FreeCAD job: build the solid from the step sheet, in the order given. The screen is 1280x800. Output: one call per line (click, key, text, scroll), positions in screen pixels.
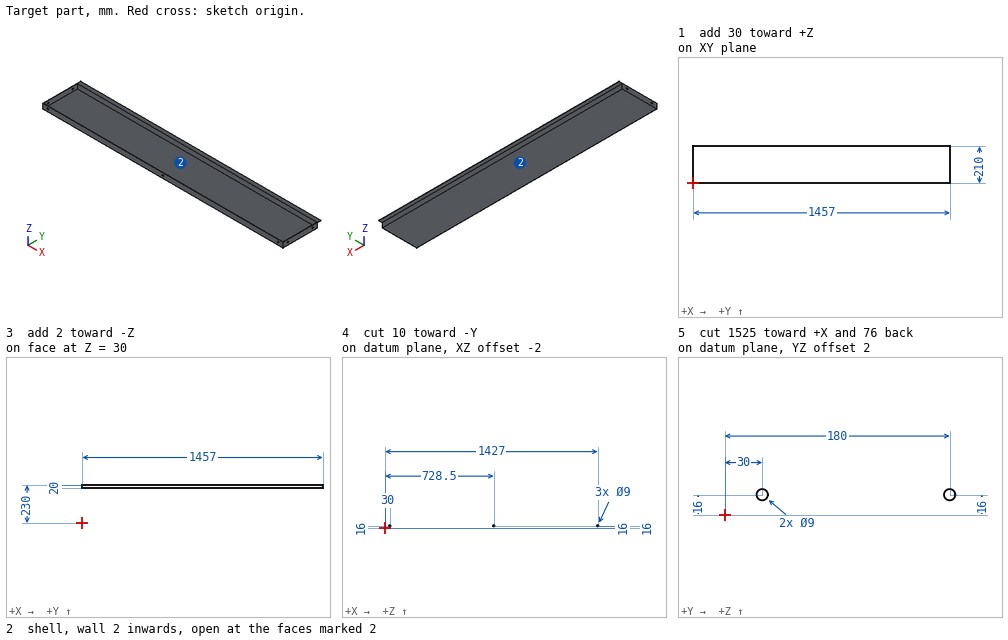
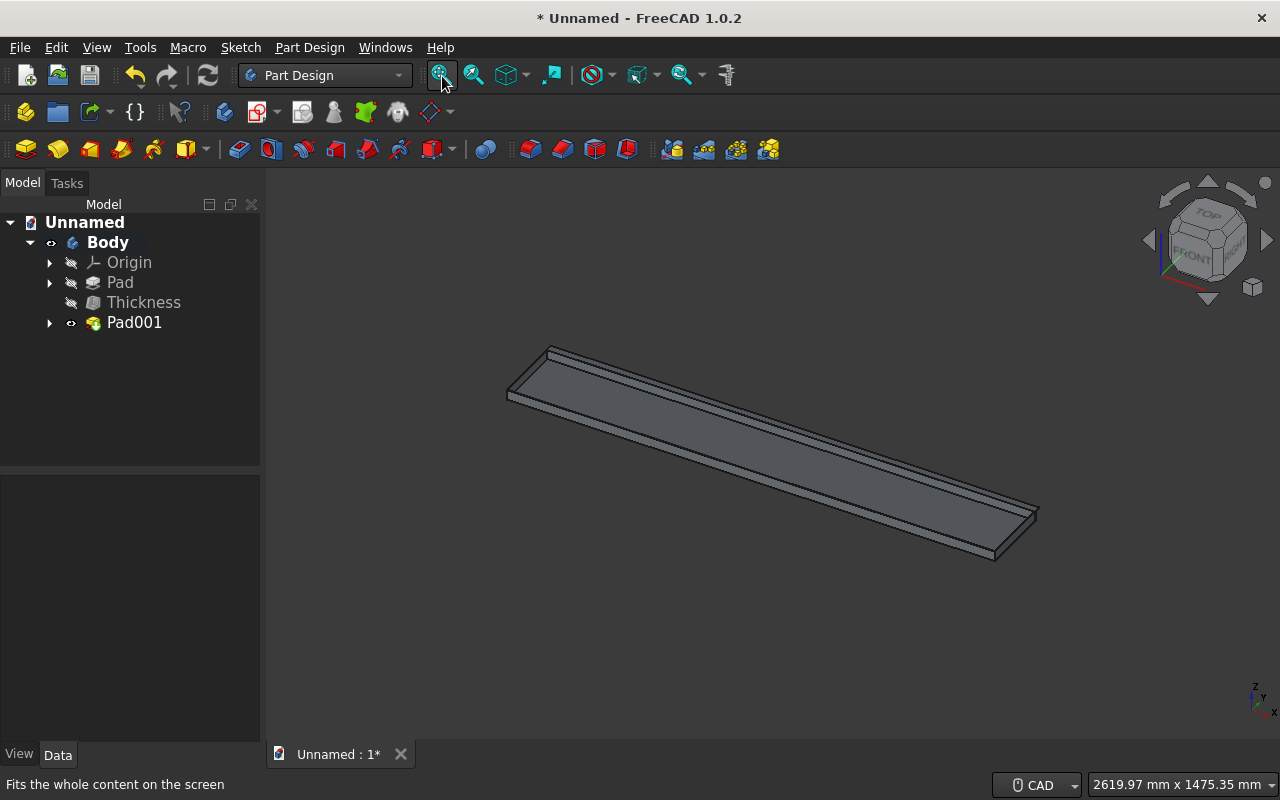
click(50, 263)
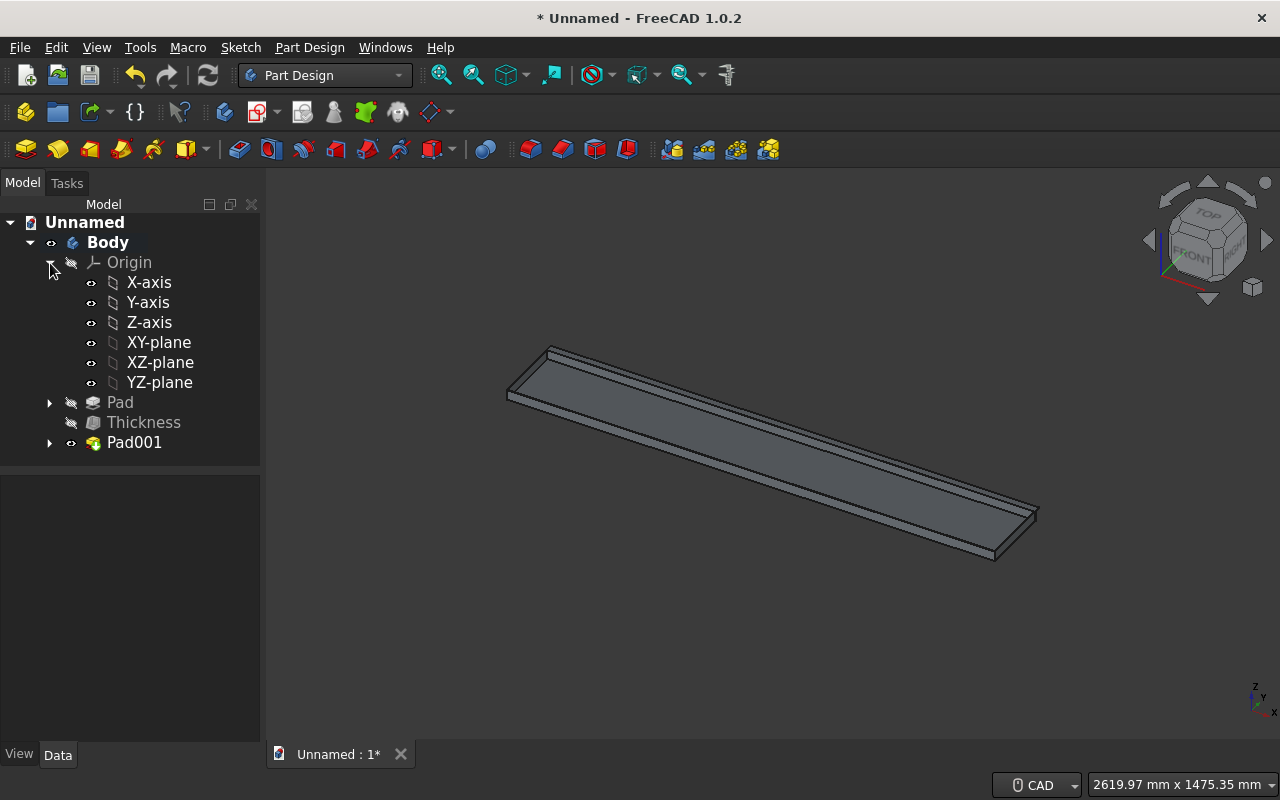
click(136, 363)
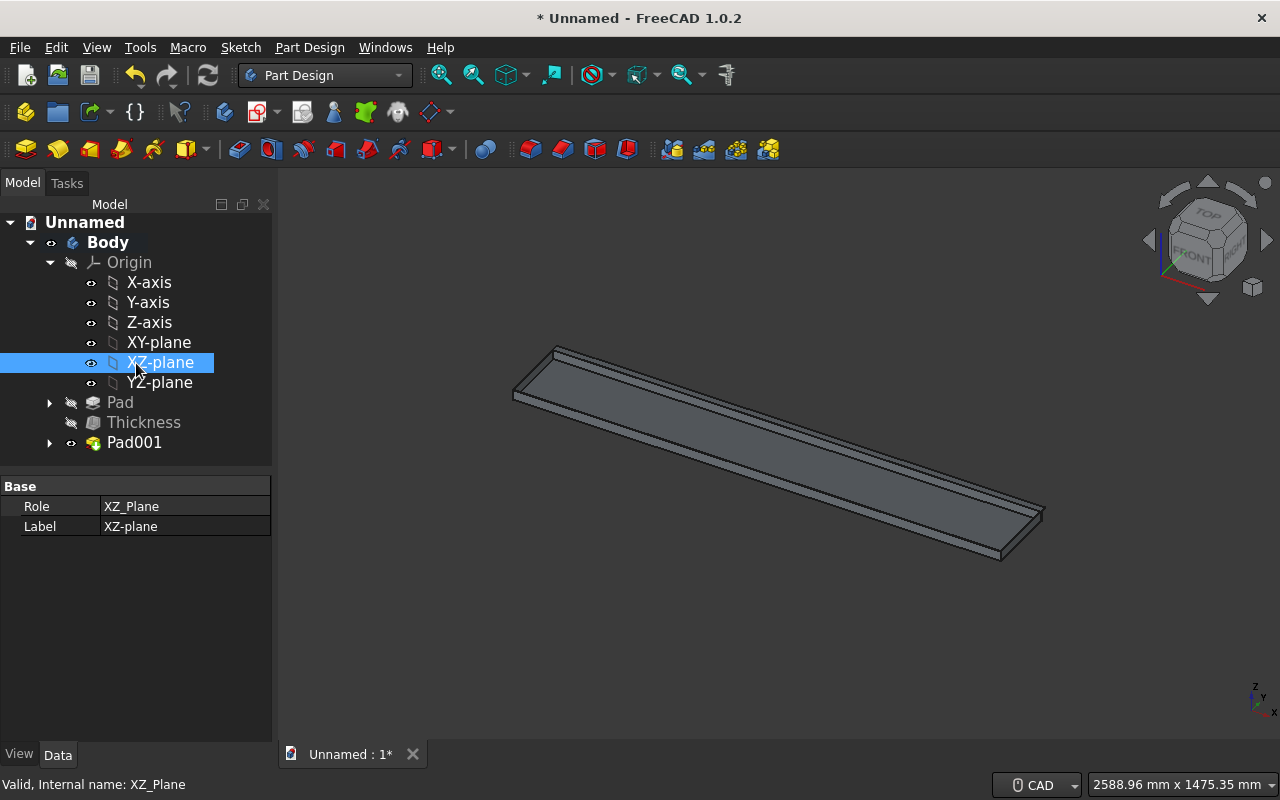
click(430, 112)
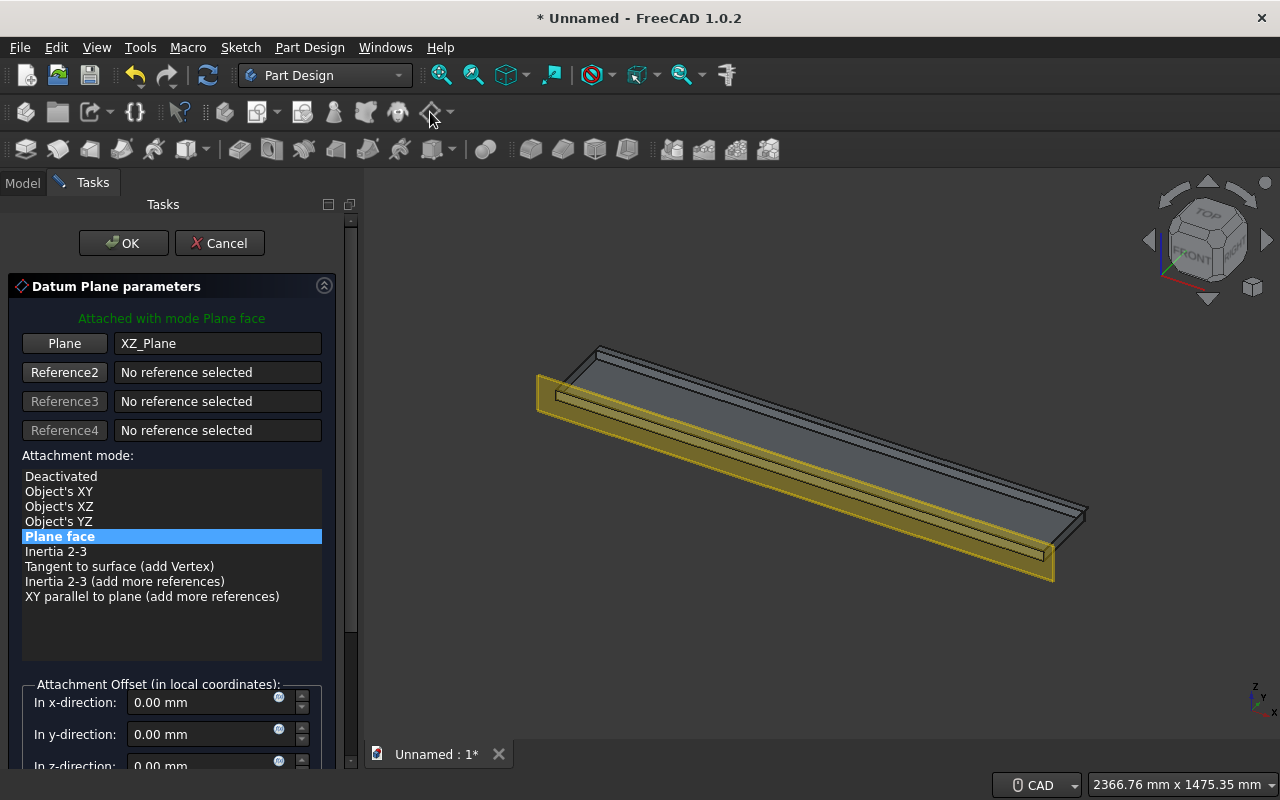
scroll(351, 491, down, 2)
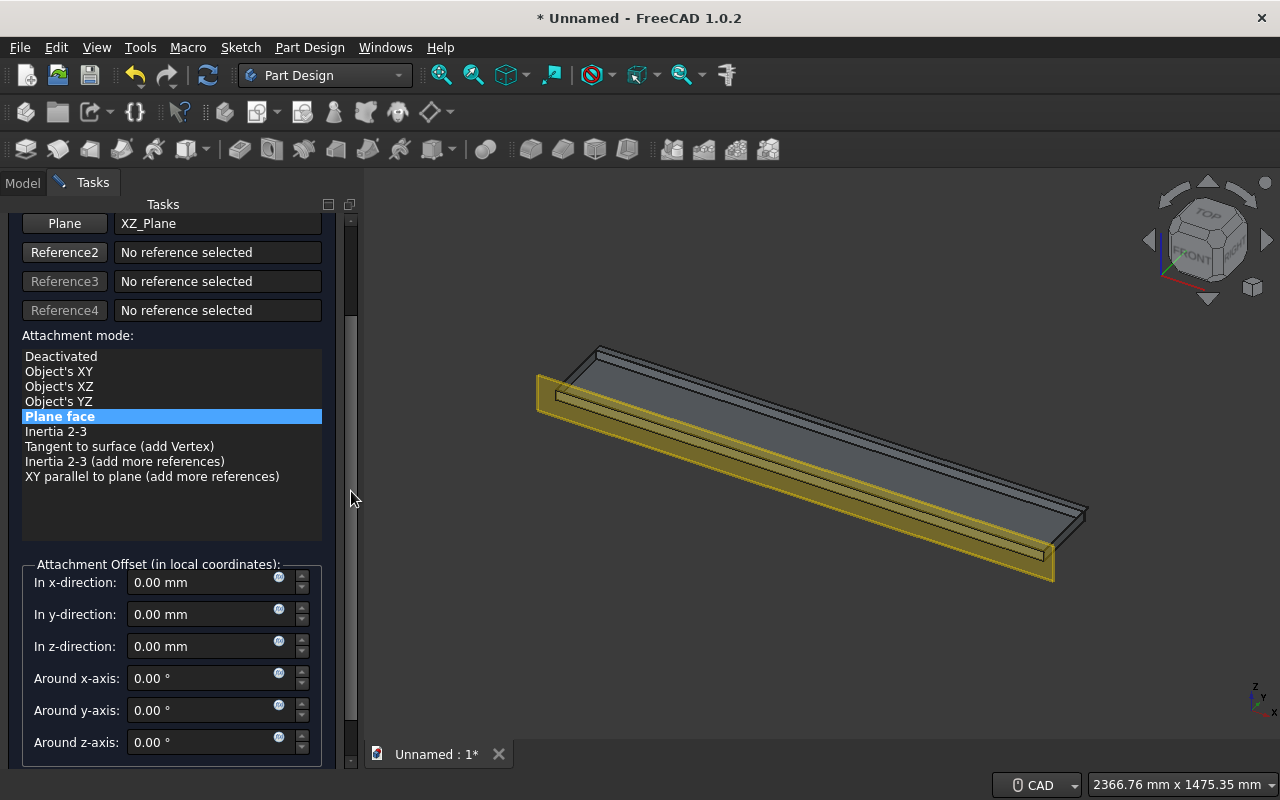
triple_click(210, 646)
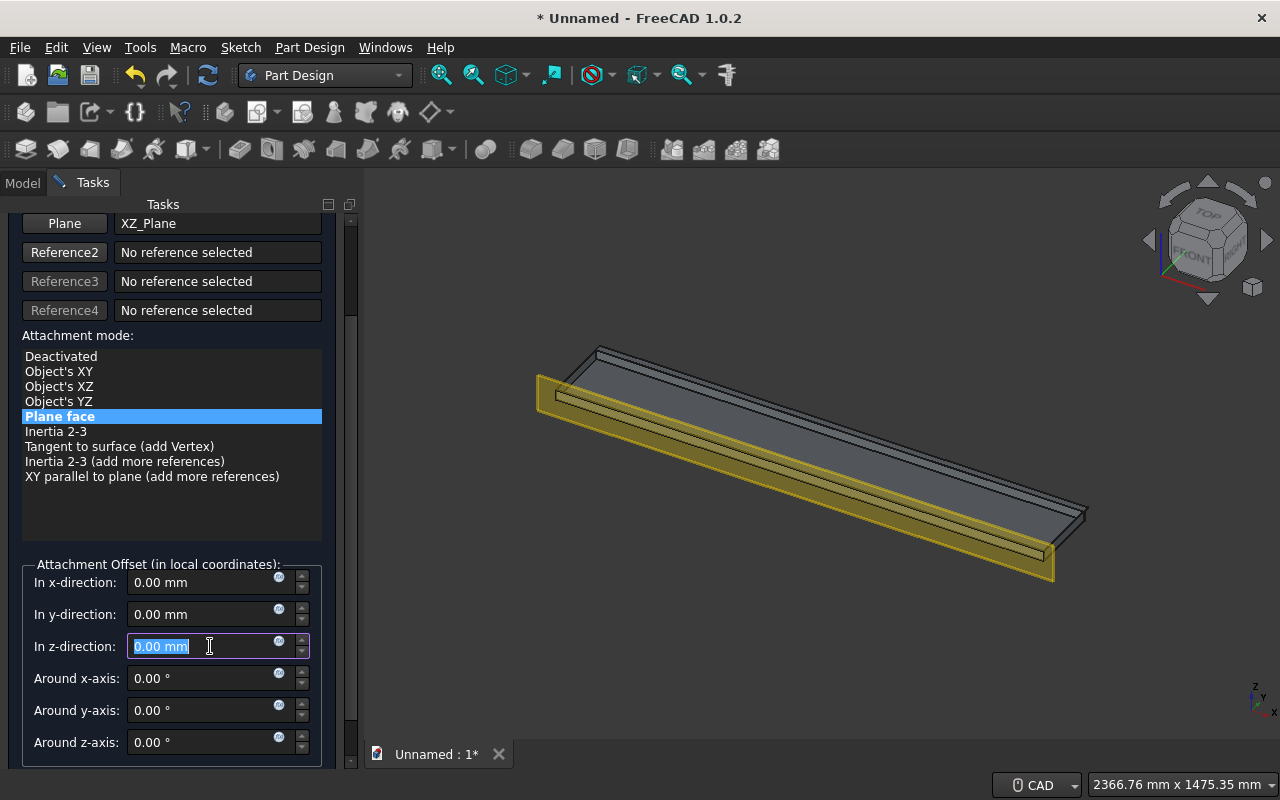
text(-2)
key(Tab)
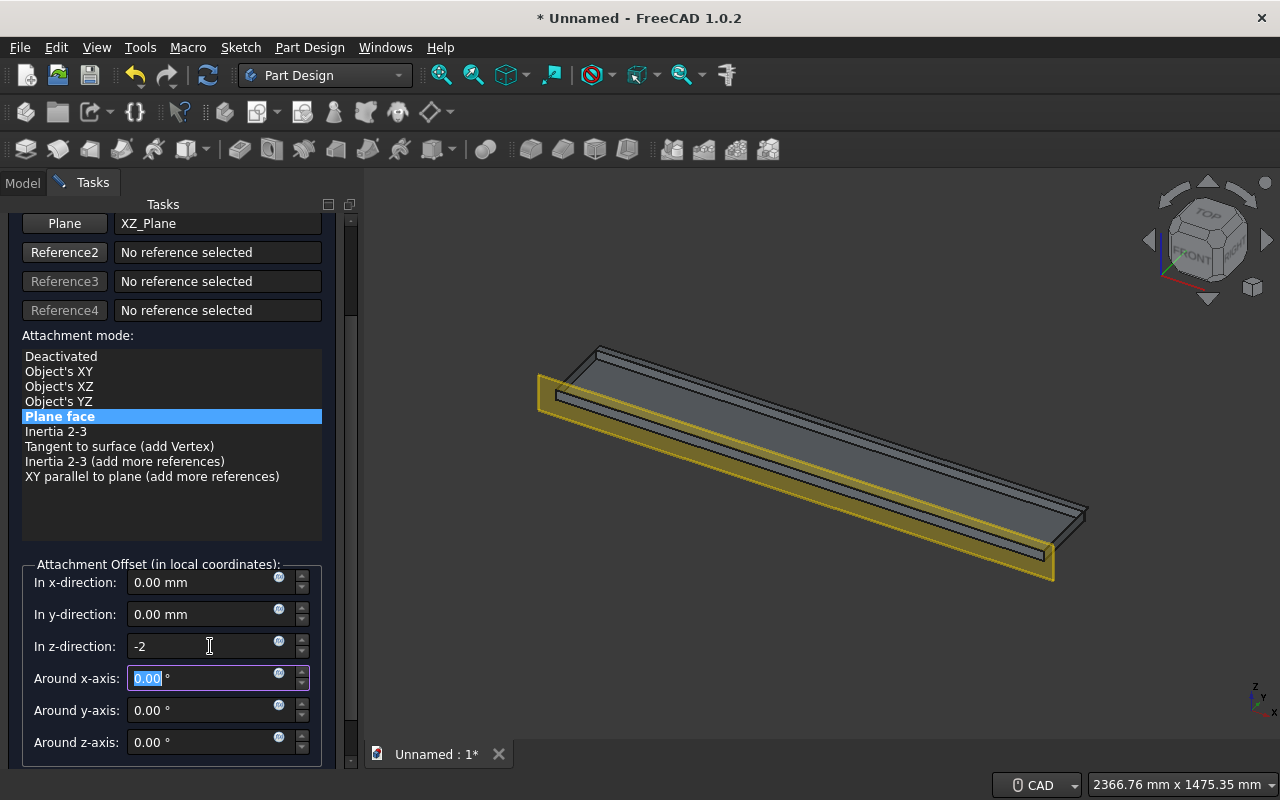
scroll(351, 491, up, 3)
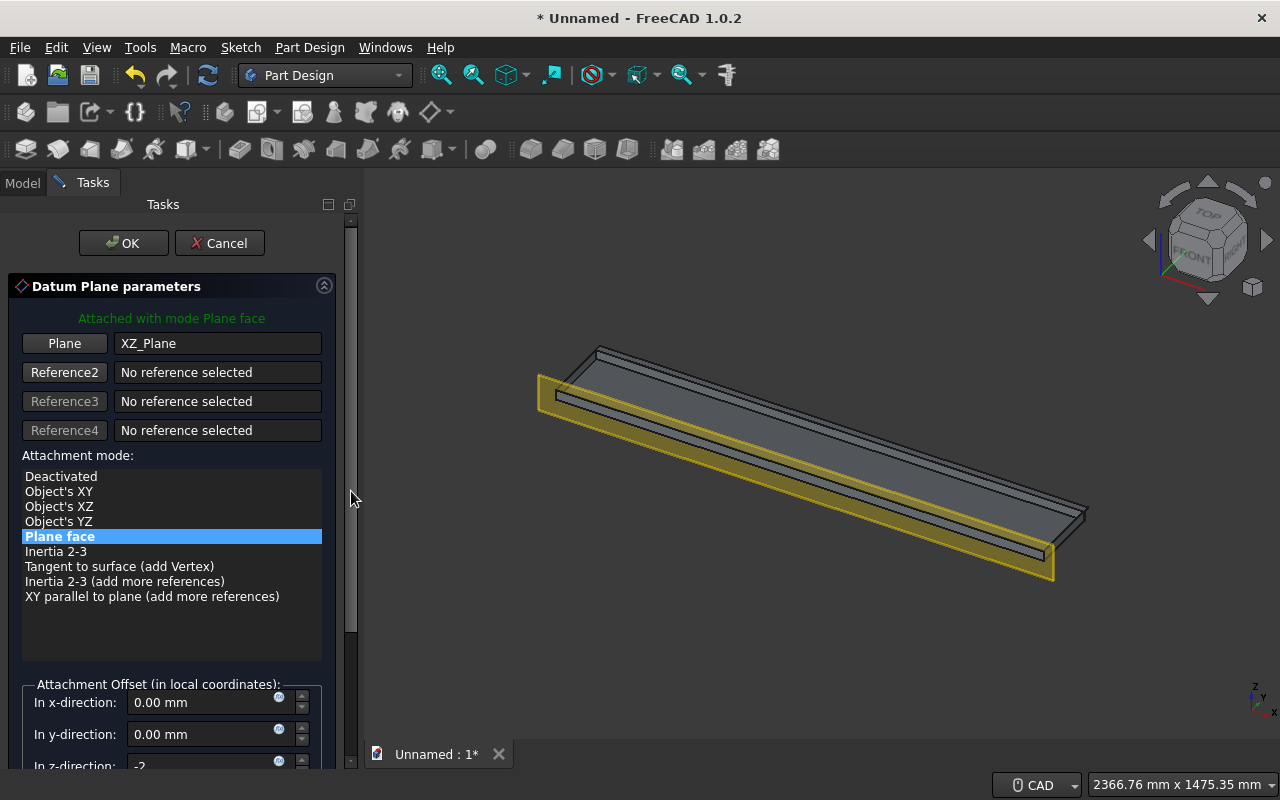
click(124, 243)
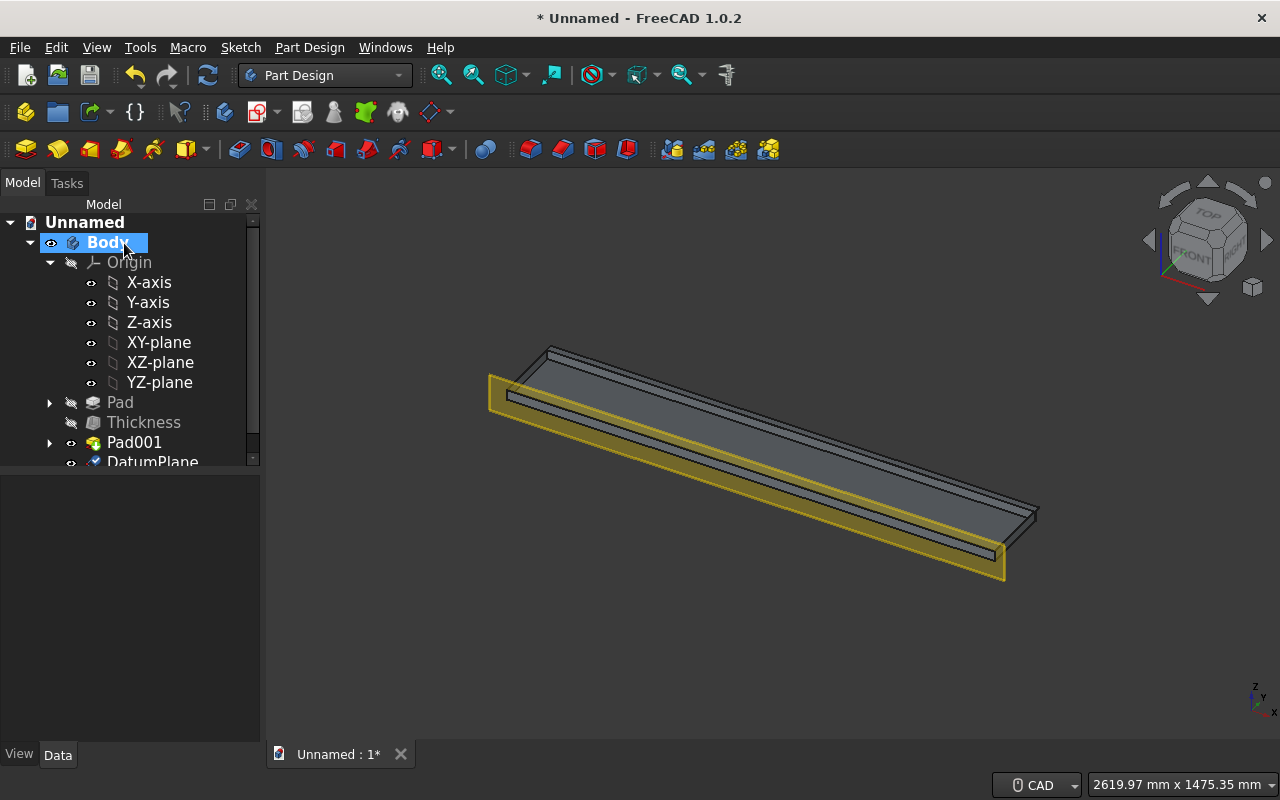
click(116, 463)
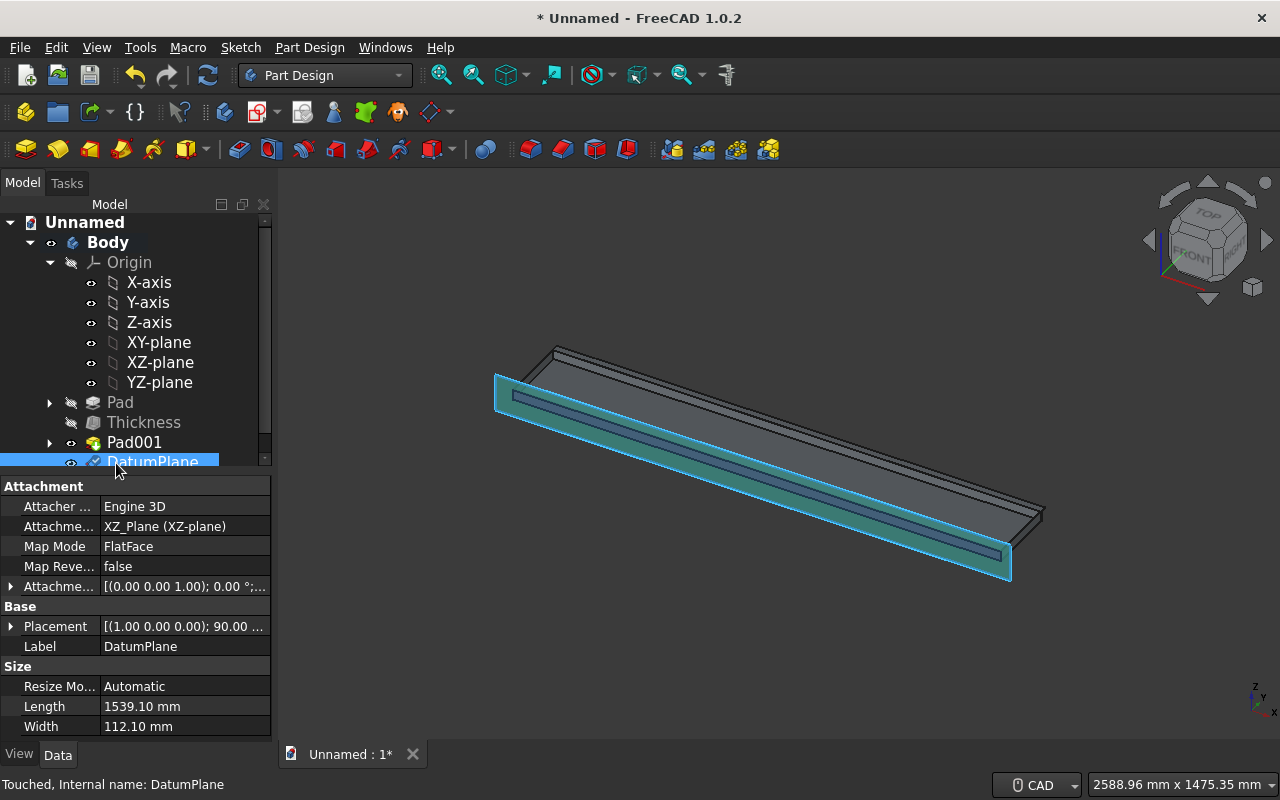
click(258, 112)